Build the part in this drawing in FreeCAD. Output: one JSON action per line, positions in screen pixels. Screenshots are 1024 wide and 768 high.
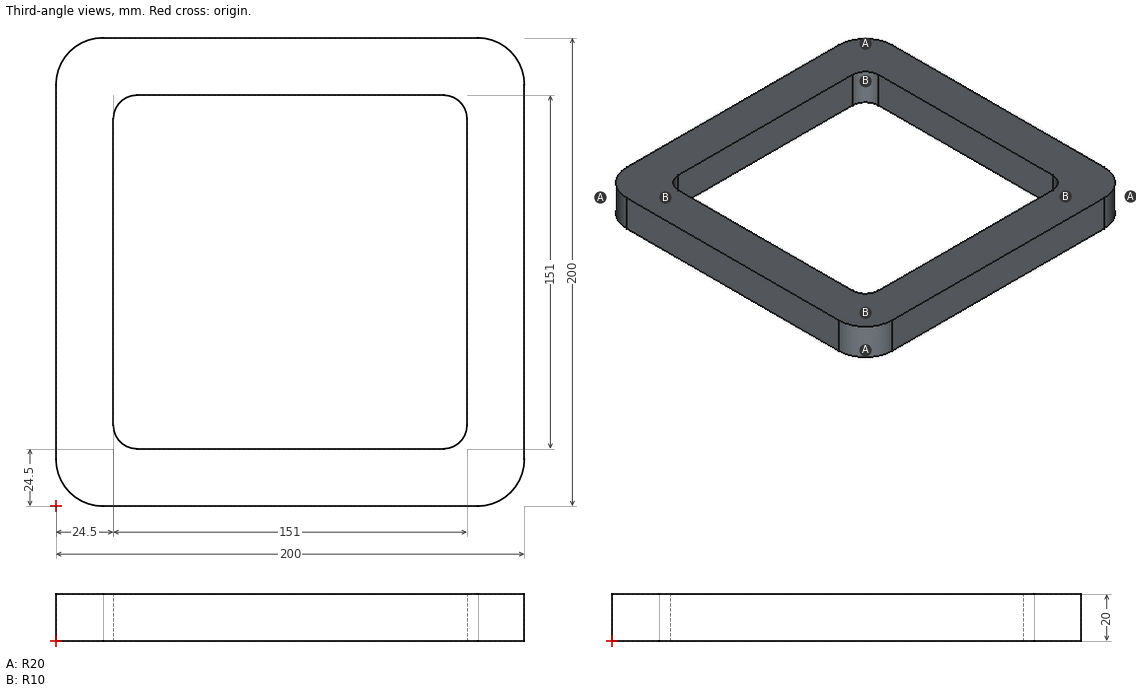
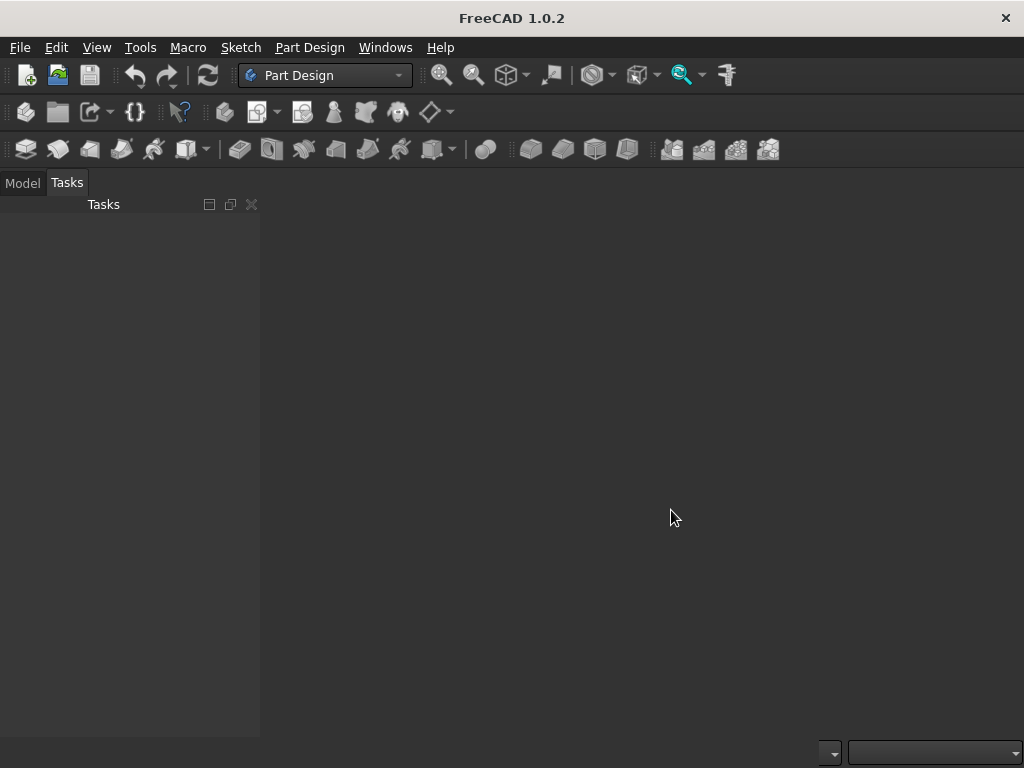
{"action": "left_click", "coordinate": [26, 76]}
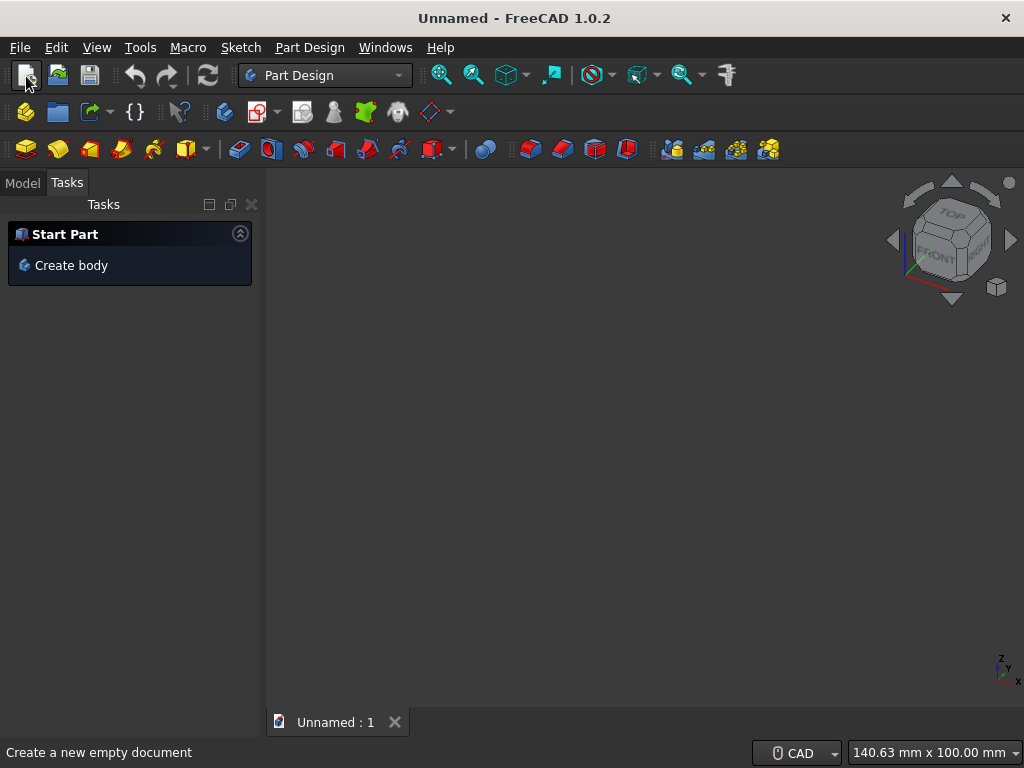
{"action": "left_click", "coordinate": [258, 112]}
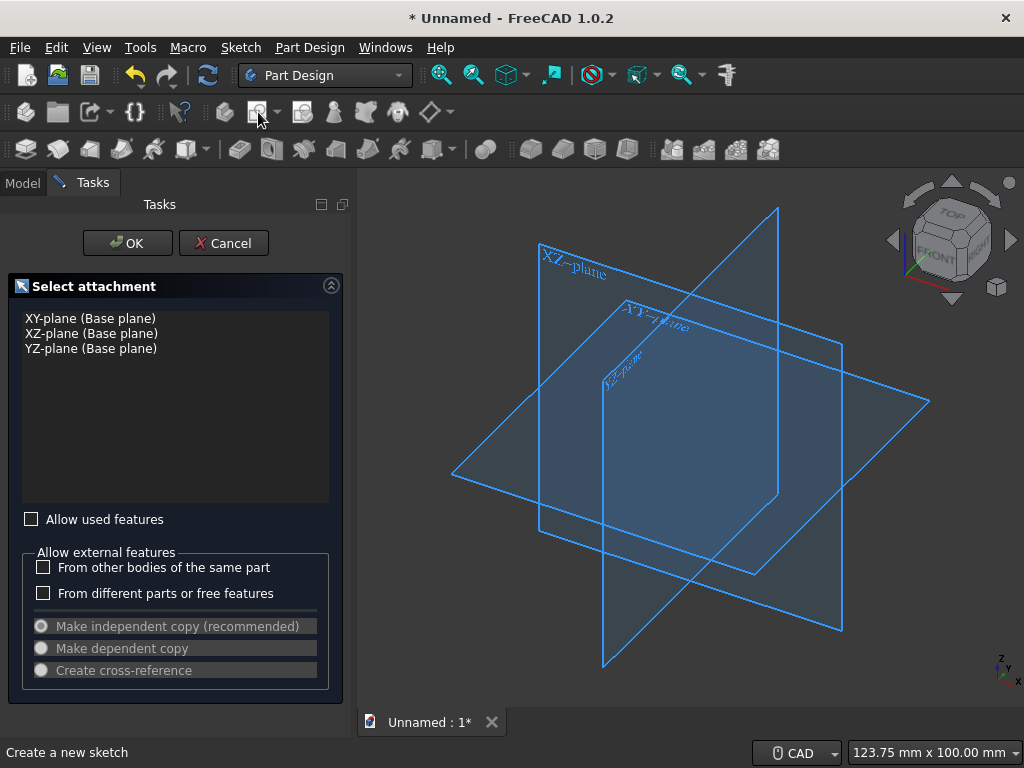
{"action": "left_click", "coordinate": [82, 318]}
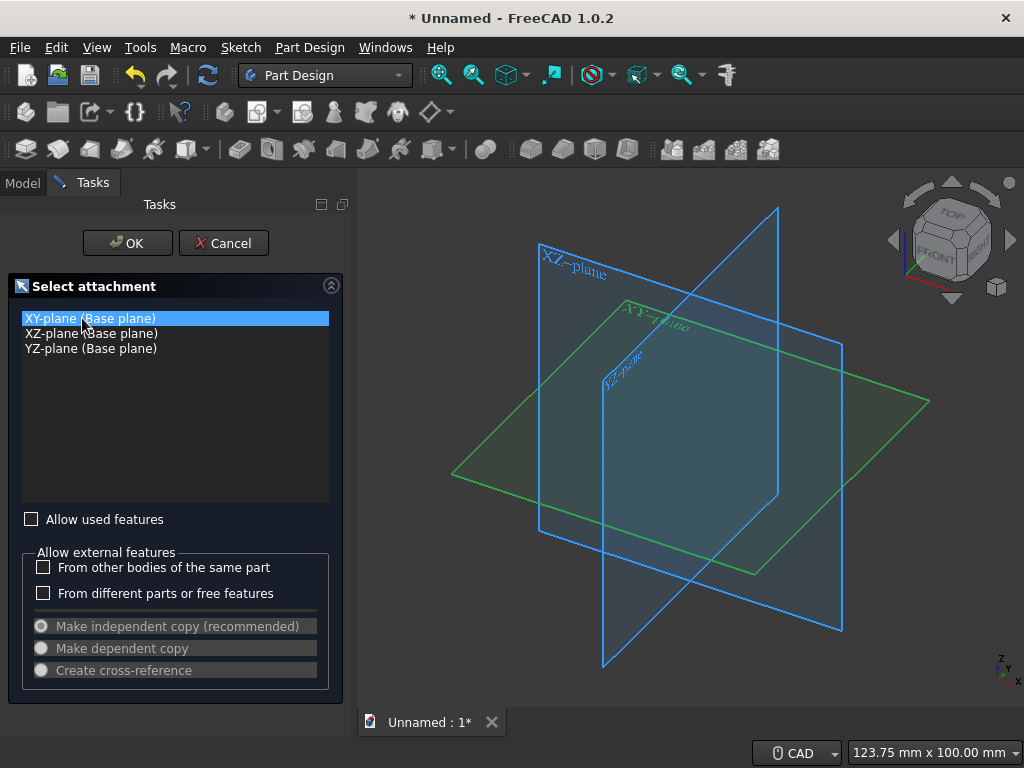
{"action": "left_click", "coordinate": [128, 243]}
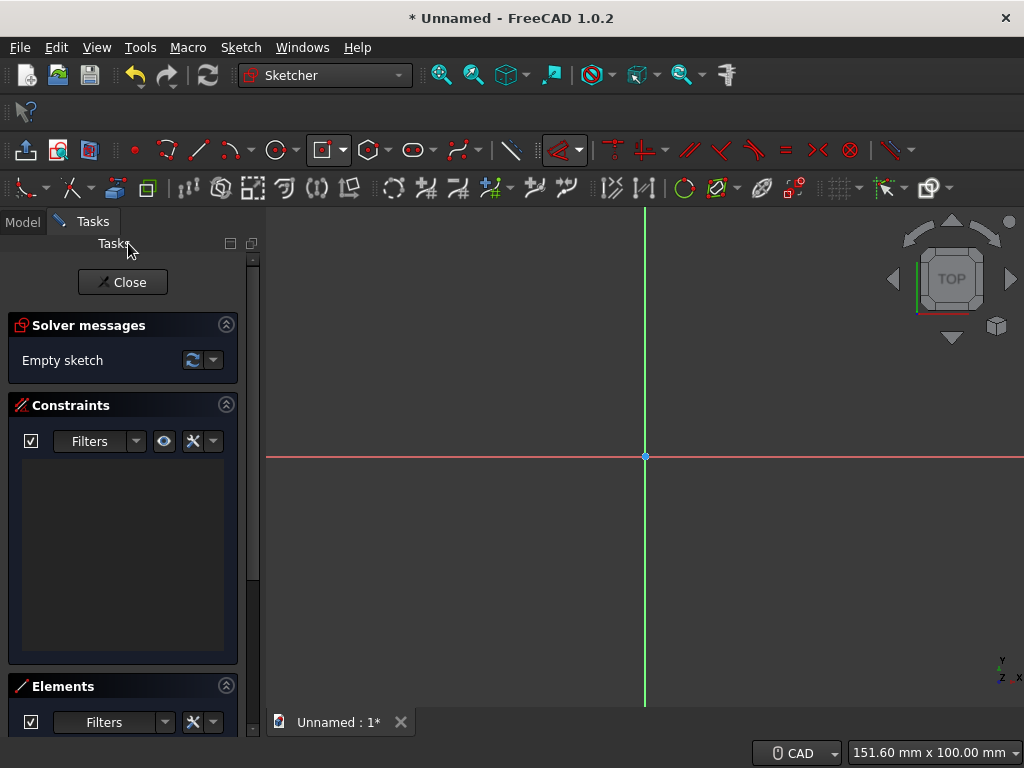
{"action": "scroll", "coordinate": [331, 673], "scroll_direction": "down", "scroll_amount": 6}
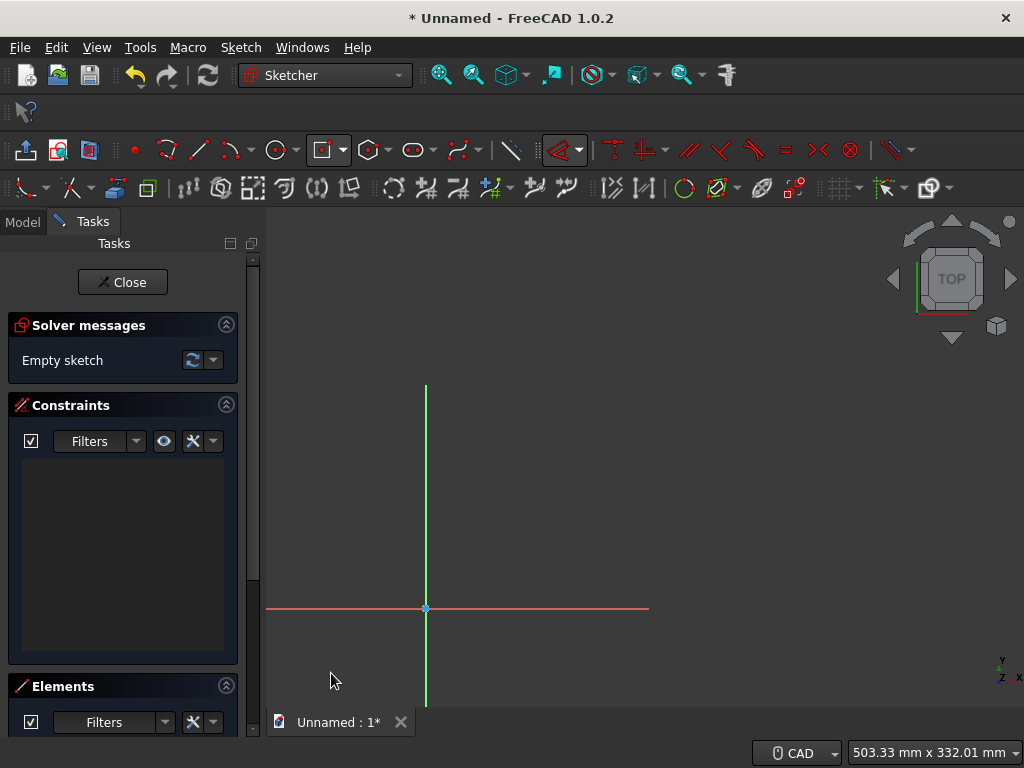
{"action": "left_click", "coordinate": [346, 150]}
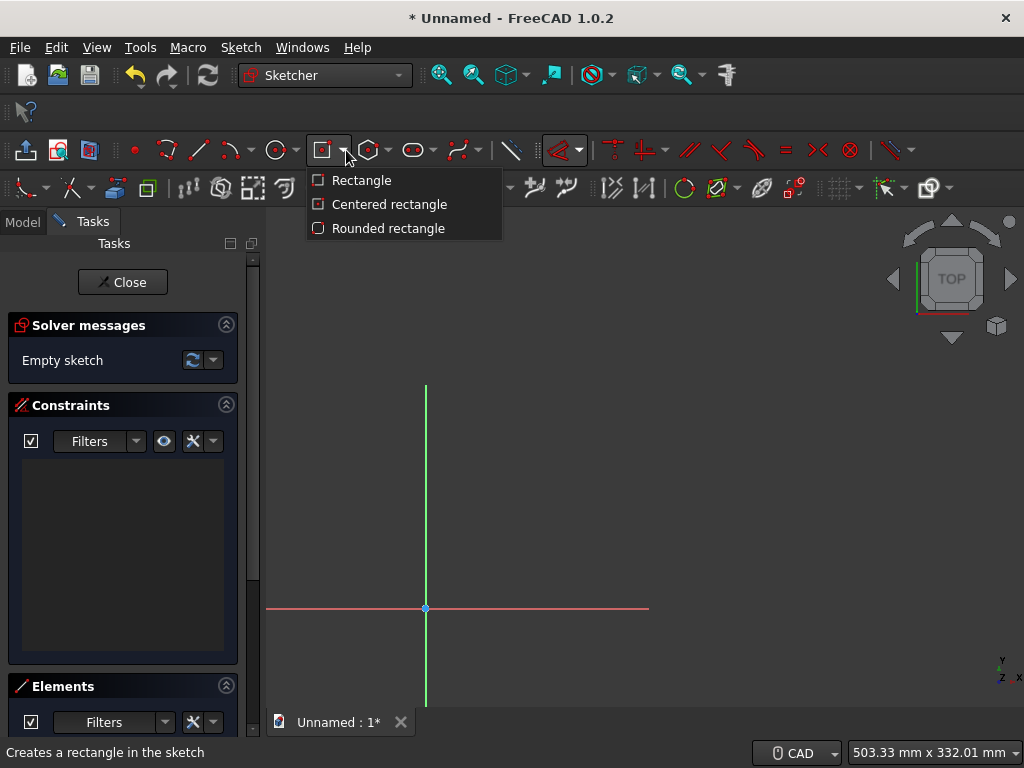
{"action": "left_click", "coordinate": [404, 180]}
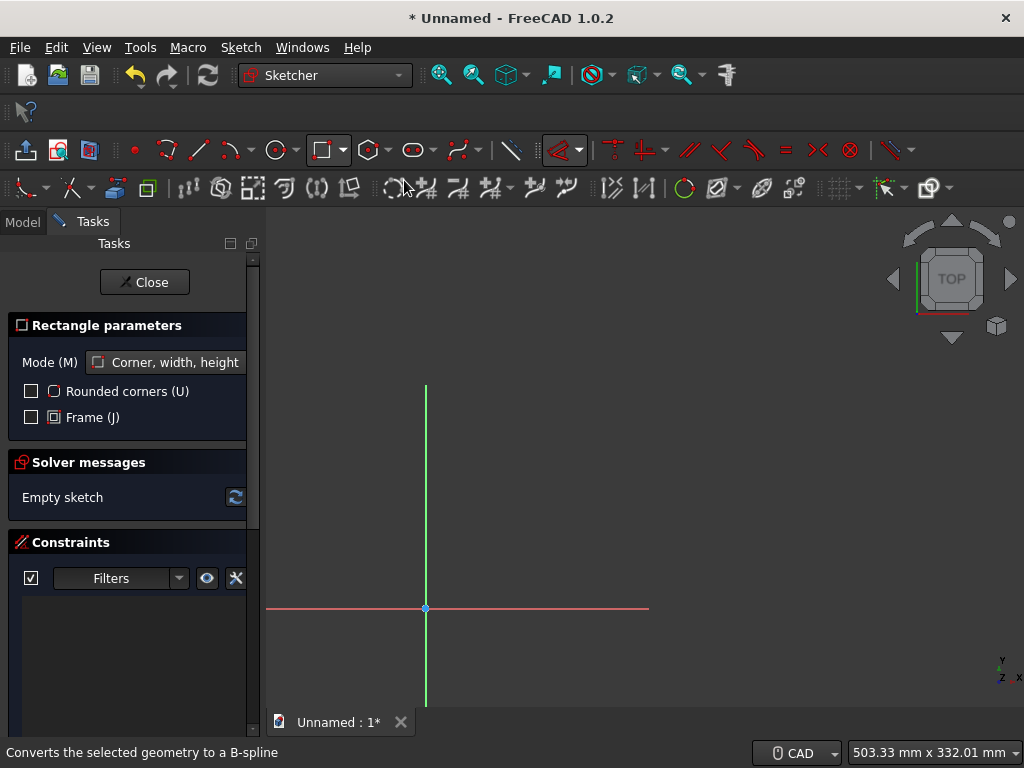
{"action": "left_click", "coordinate": [426, 609]}
{"action": "mouse_move", "coordinate": [727, 307]}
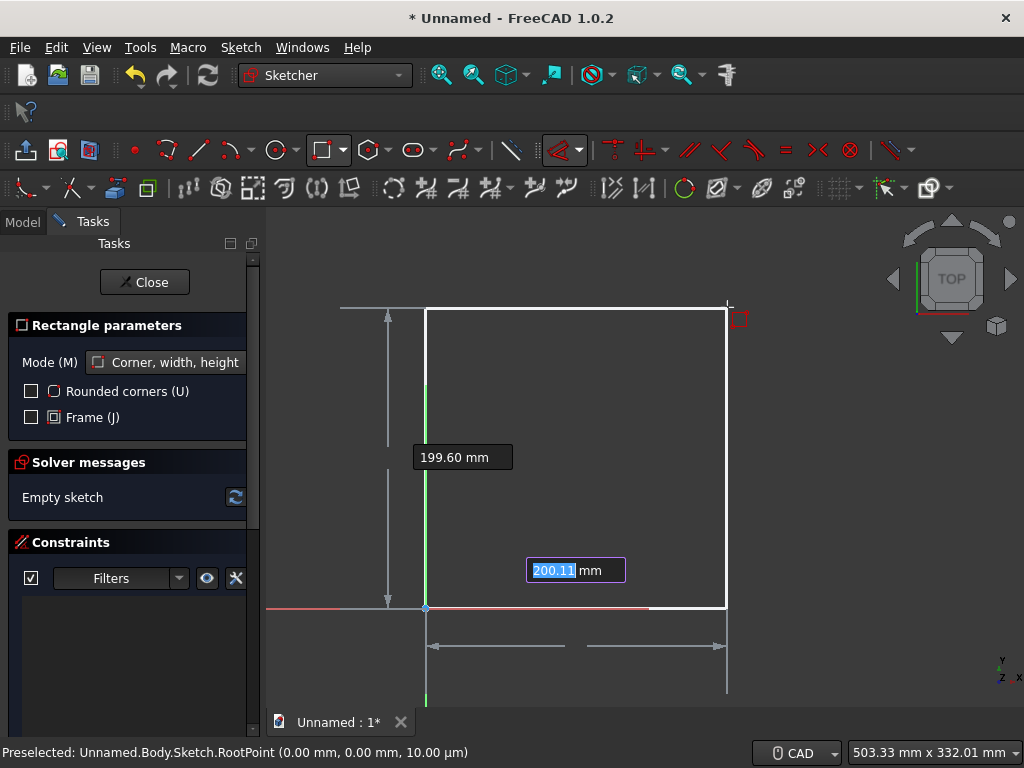
{"action": "type", "text": "200"}
{"action": "key", "text": "Tab"}
{"action": "type", "text": "200"}
{"action": "key", "text": "Return"}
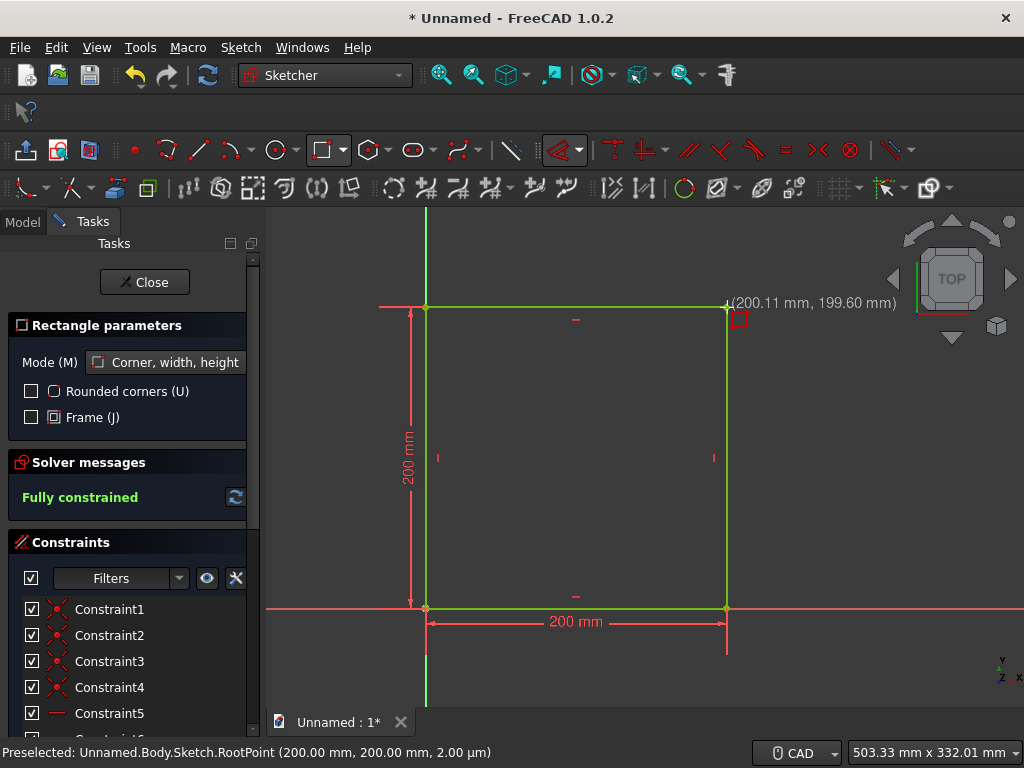
{"action": "left_click", "coordinate": [463, 344]}
{"action": "mouse_move", "coordinate": [690, 572]}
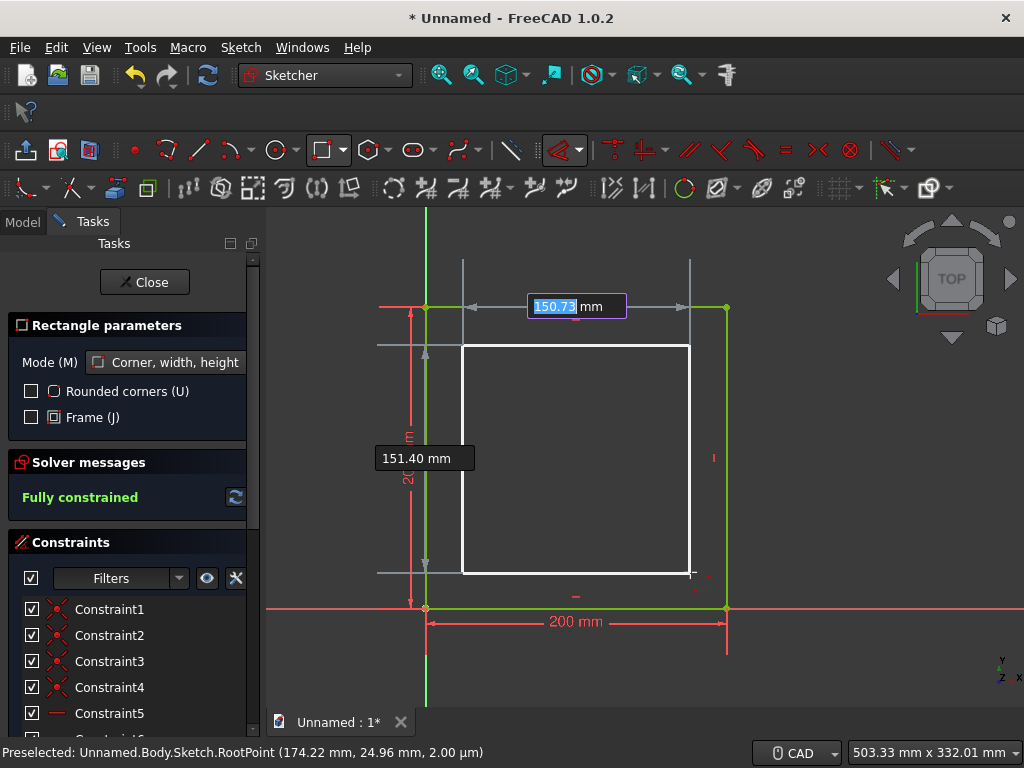
{"action": "type", "text": "151"}
{"action": "key", "text": "Tab"}
{"action": "type", "text": "151"}
{"action": "key", "text": "Return"}
{"action": "key", "text": "Escape"}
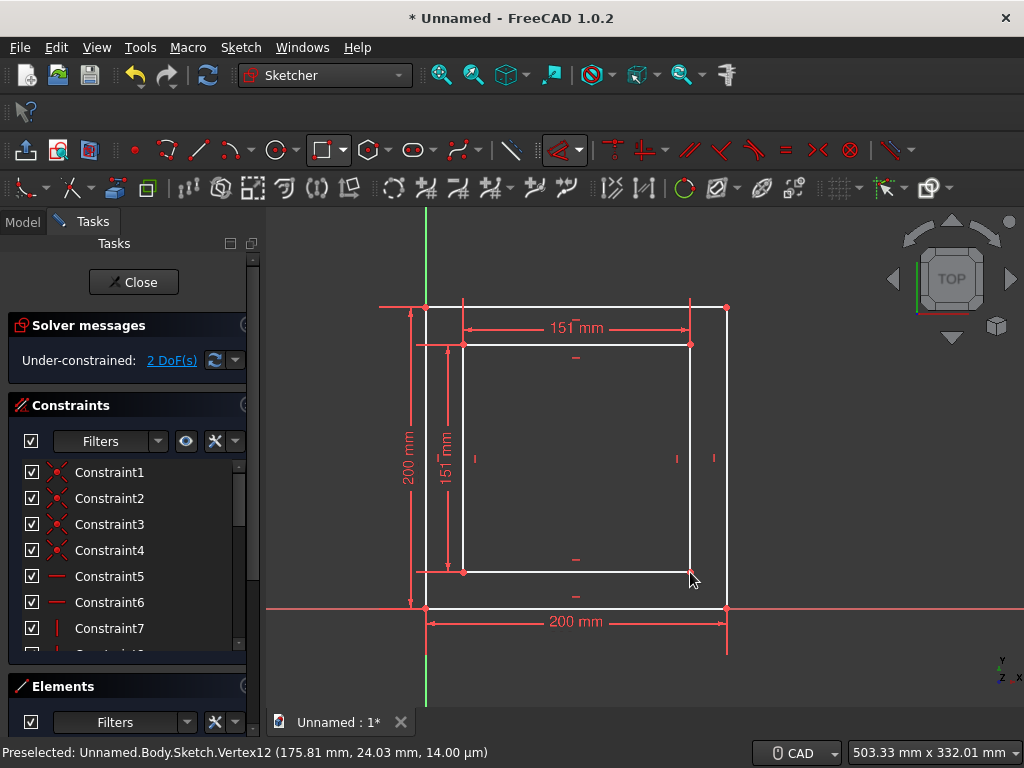
{"action": "key", "text": "d"}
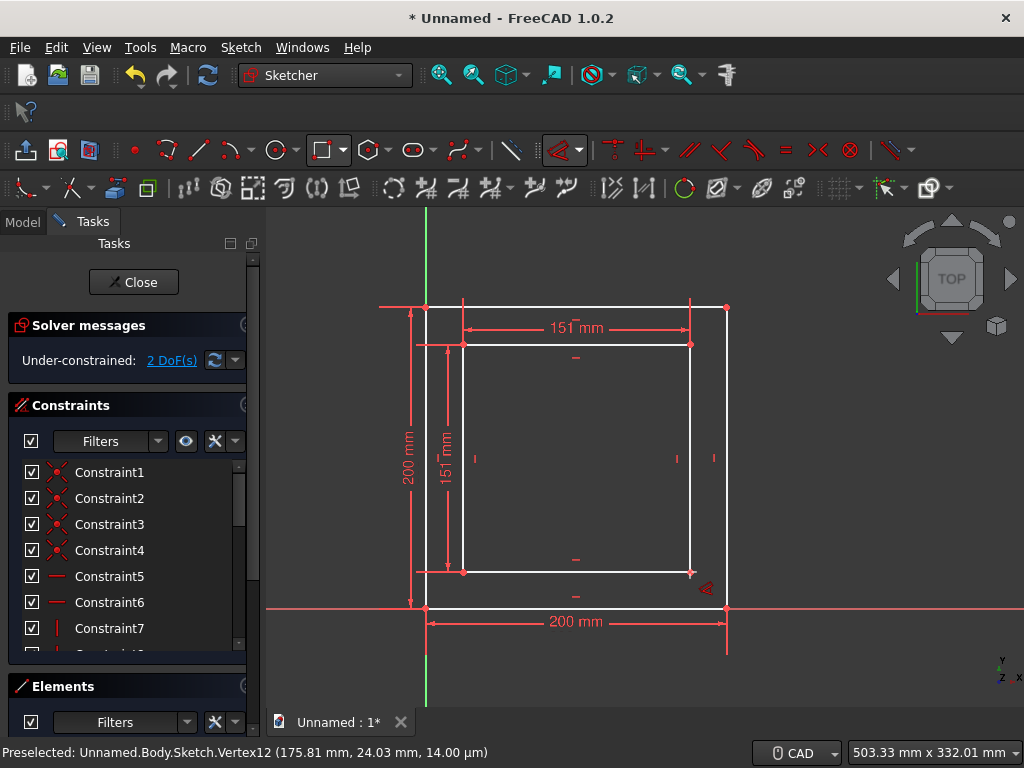
{"action": "left_click", "coordinate": [463, 345]}
{"action": "left_click", "coordinate": [444, 643]}